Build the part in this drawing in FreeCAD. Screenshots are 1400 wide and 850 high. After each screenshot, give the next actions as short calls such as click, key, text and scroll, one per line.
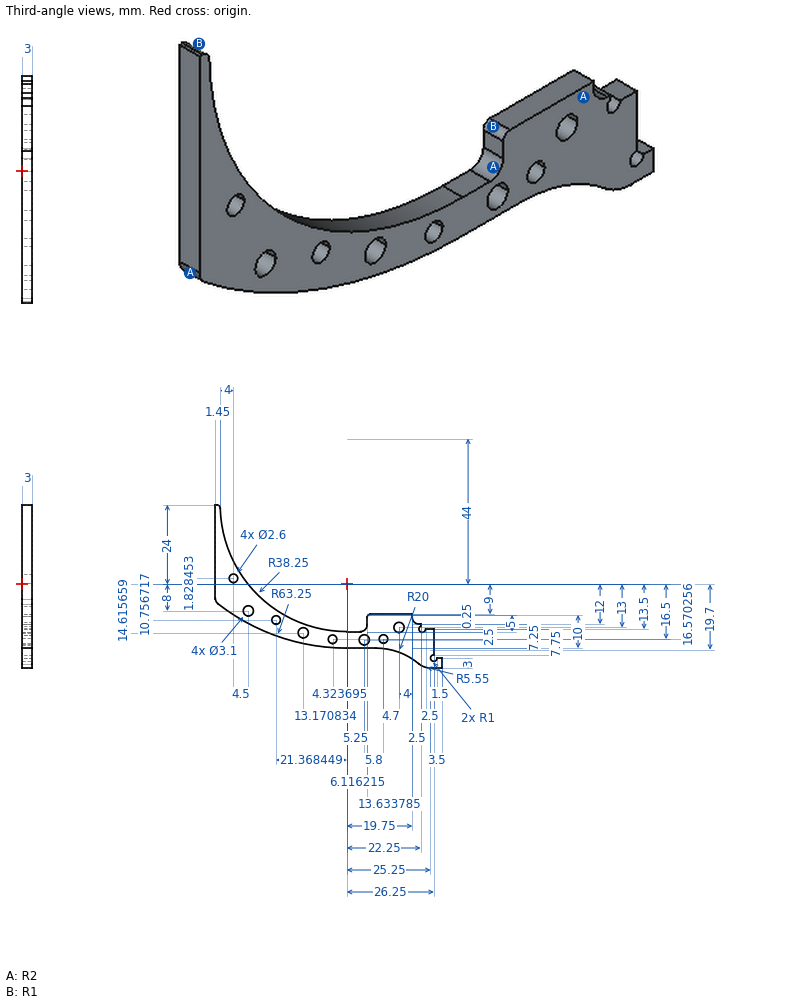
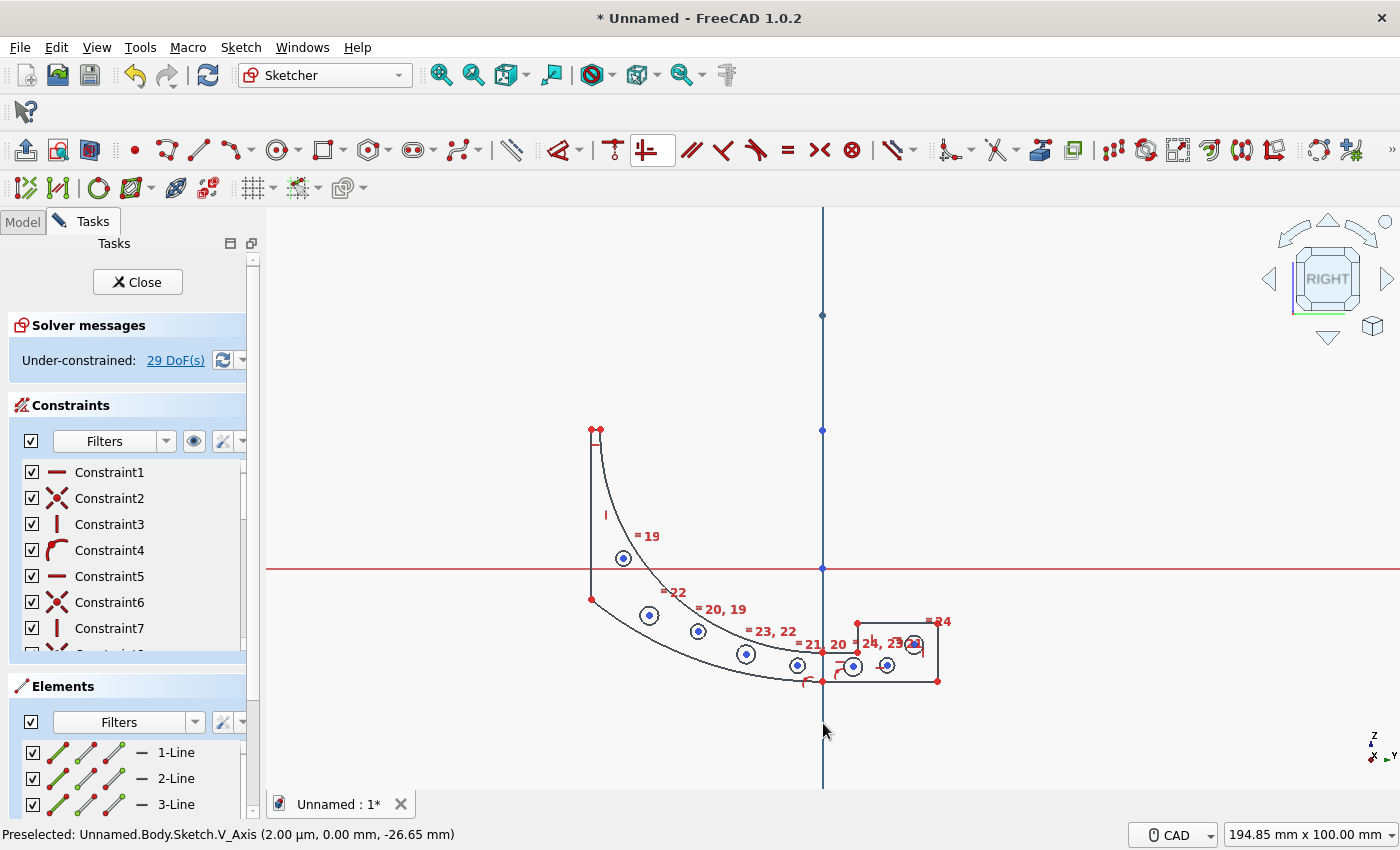
key(c)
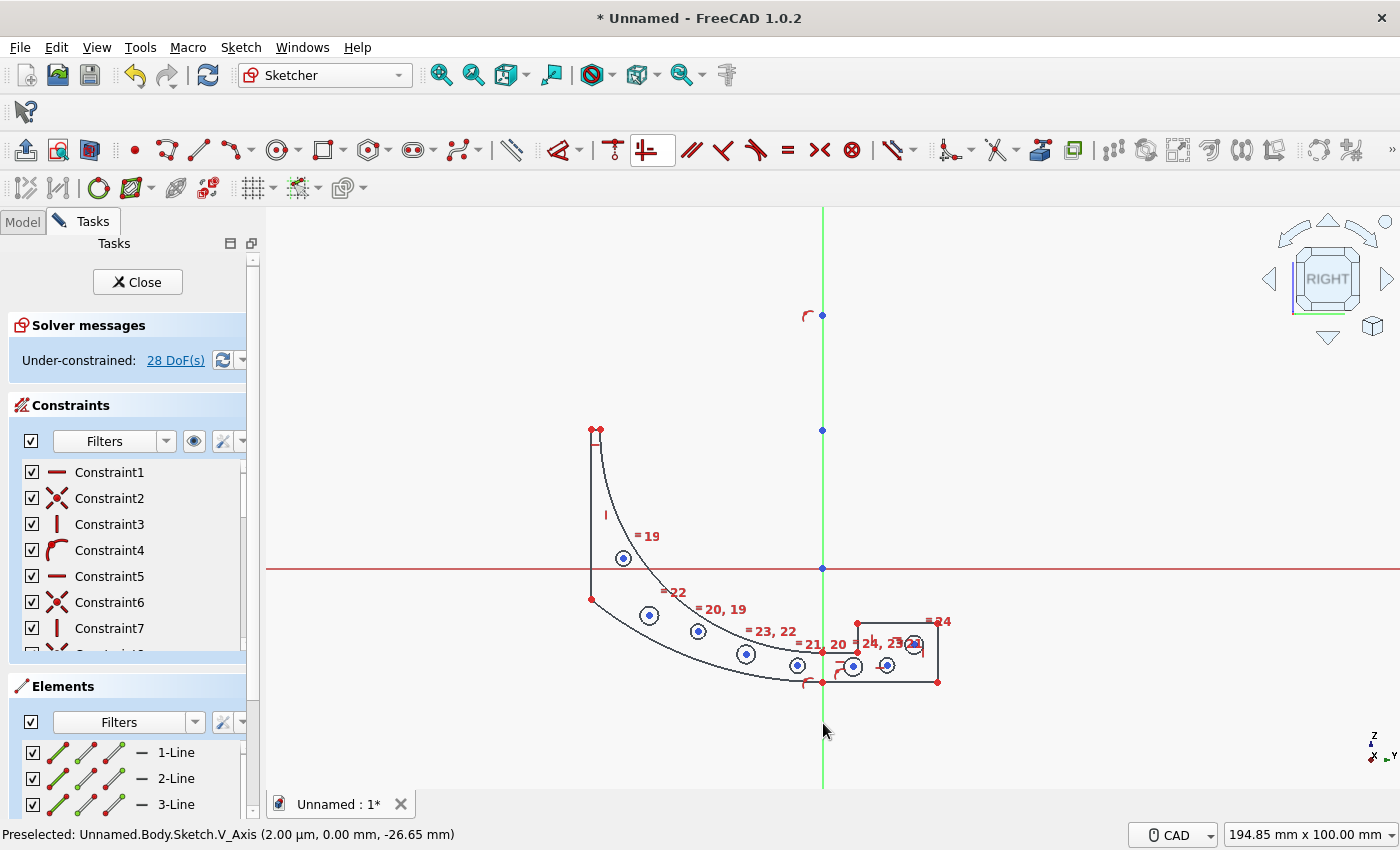
click(823, 430)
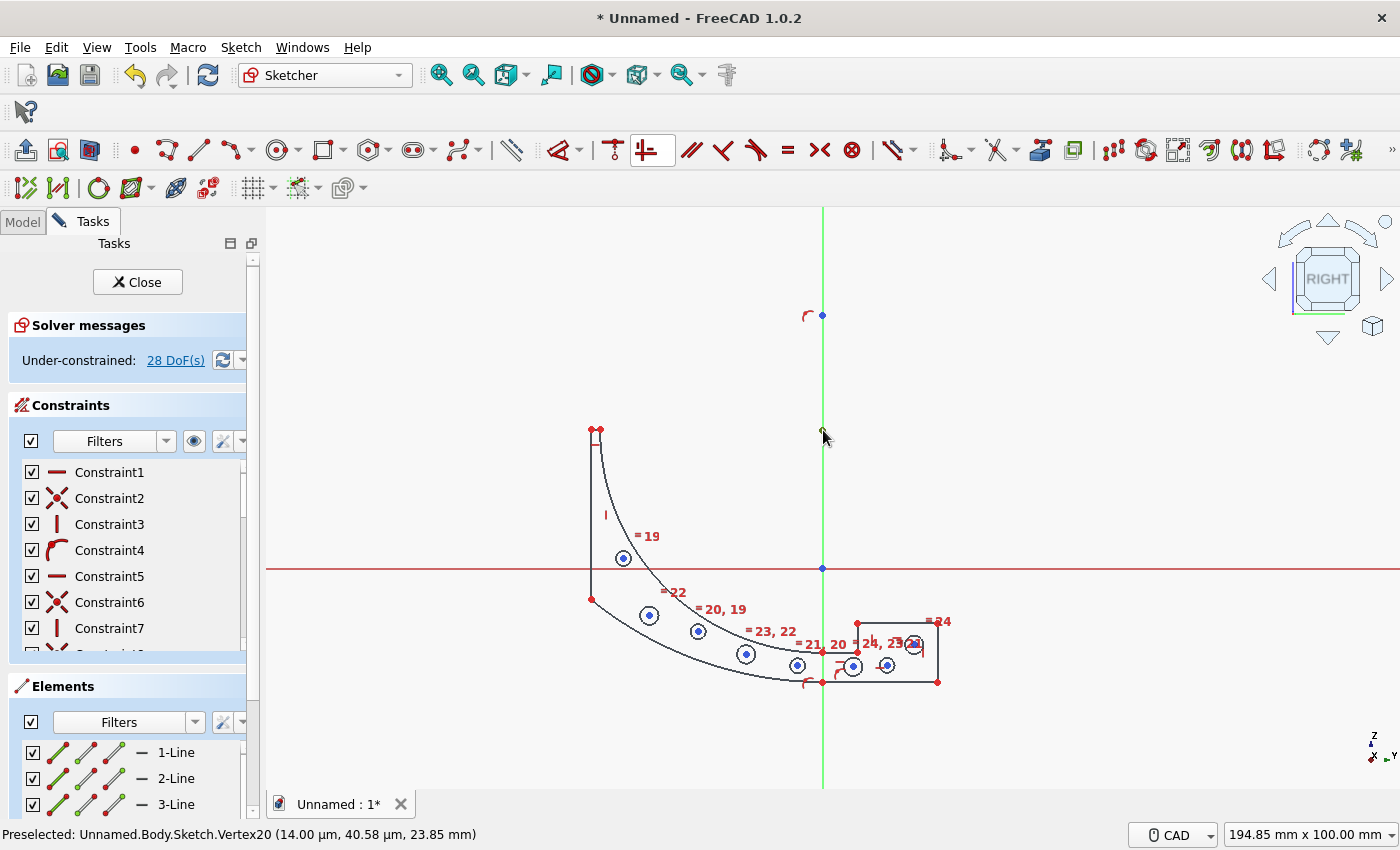
click(823, 723)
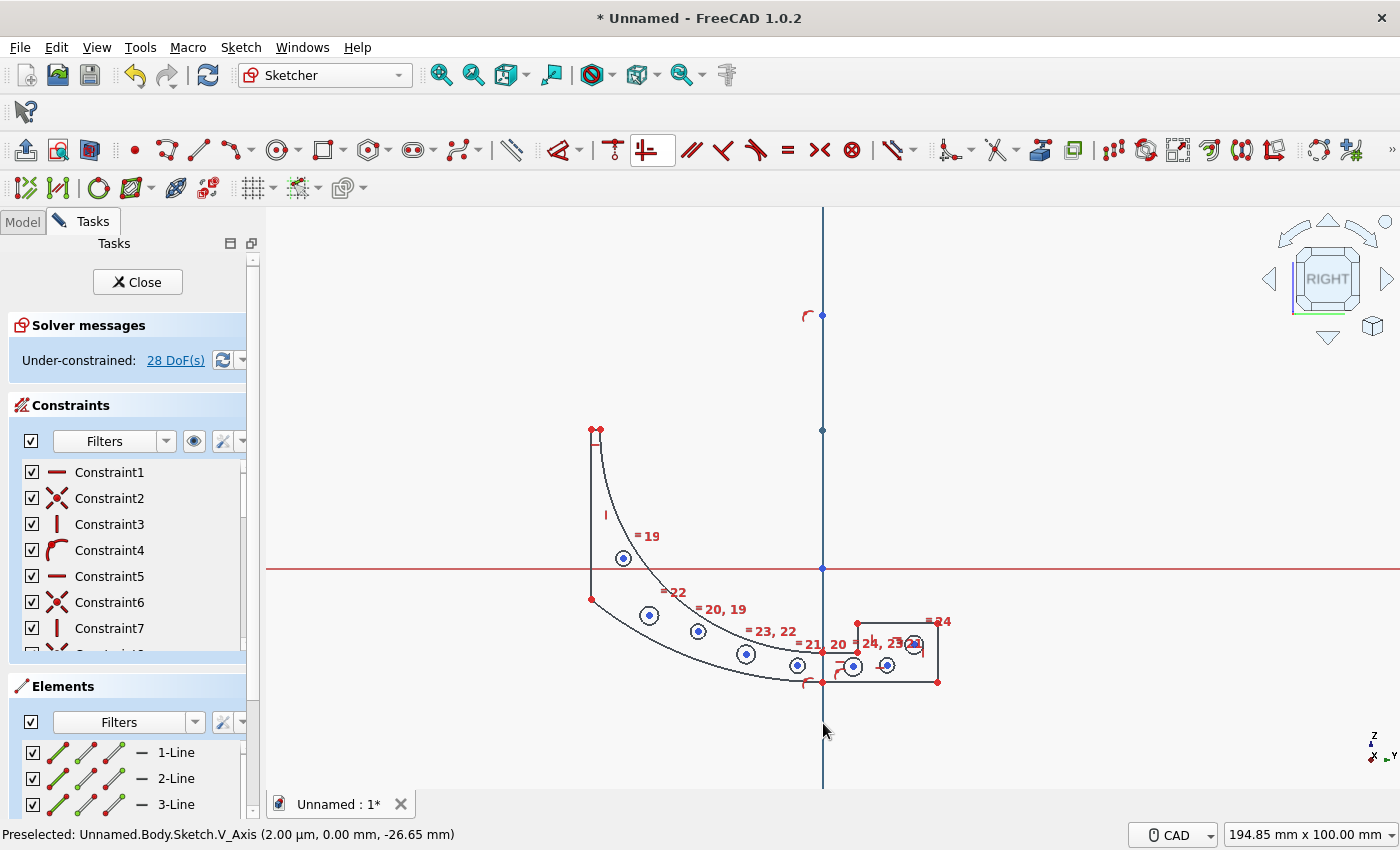
key(c)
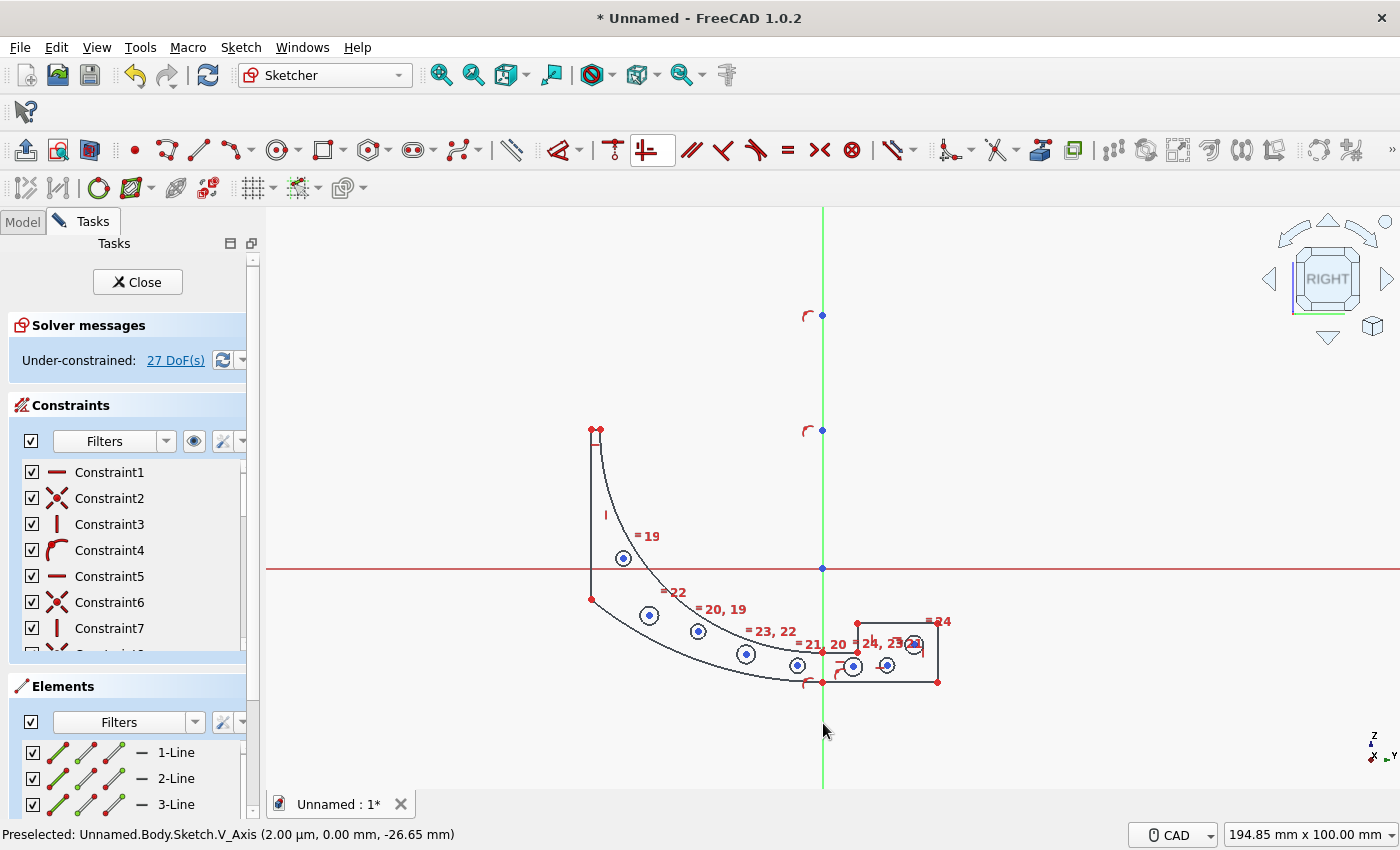
click(558, 150)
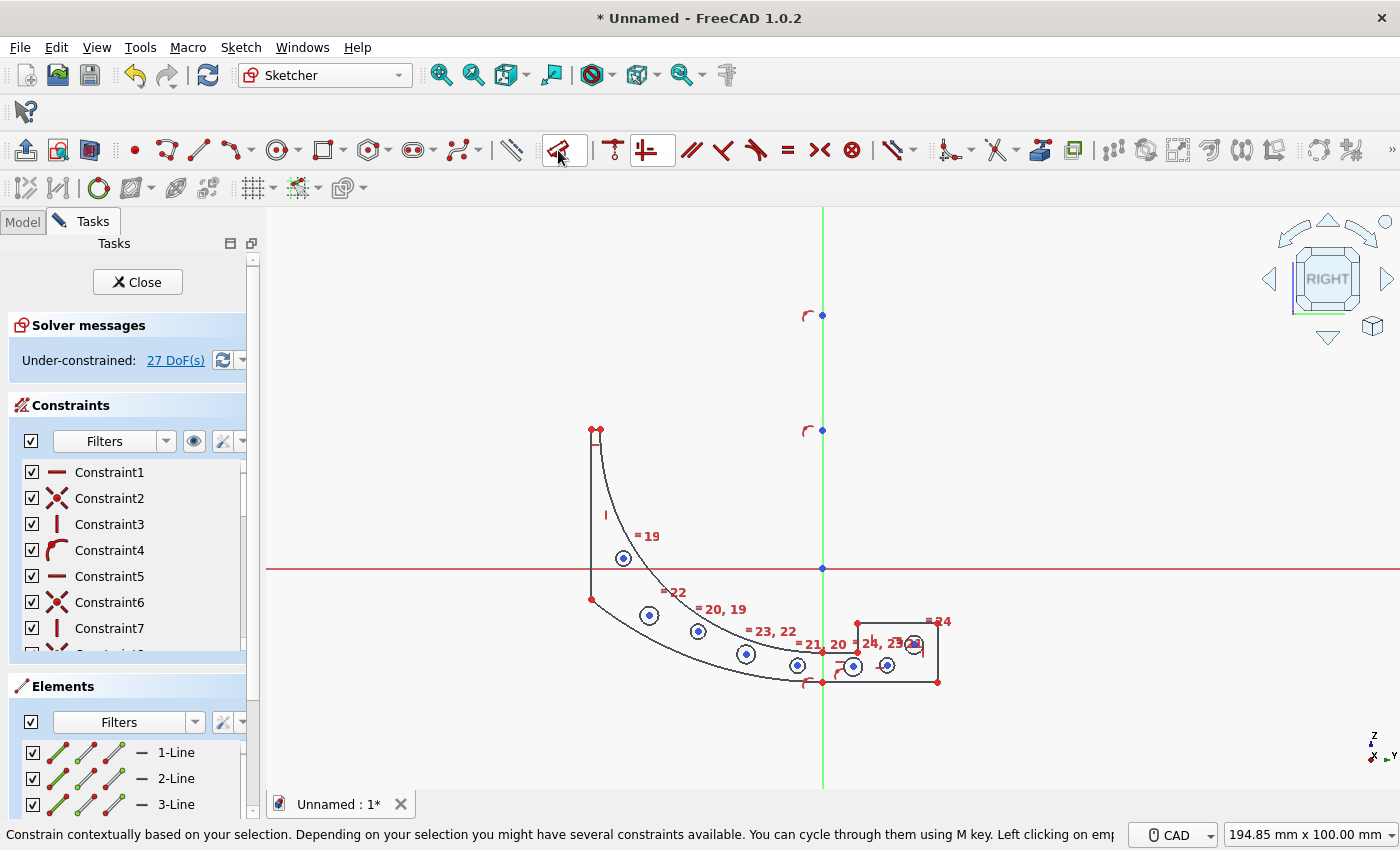
click(654, 641)
click(639, 669)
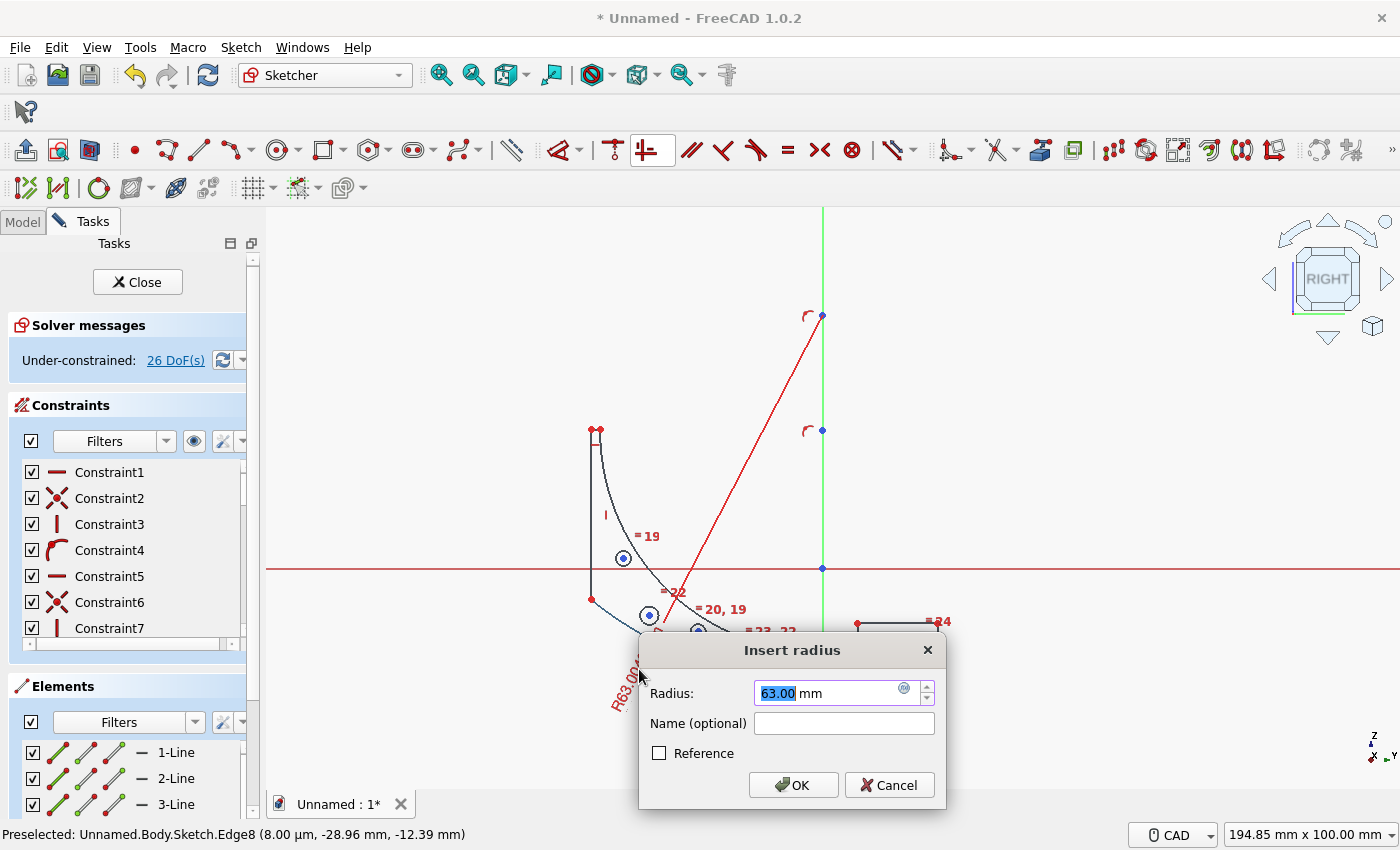
text(63.25)
key(Return)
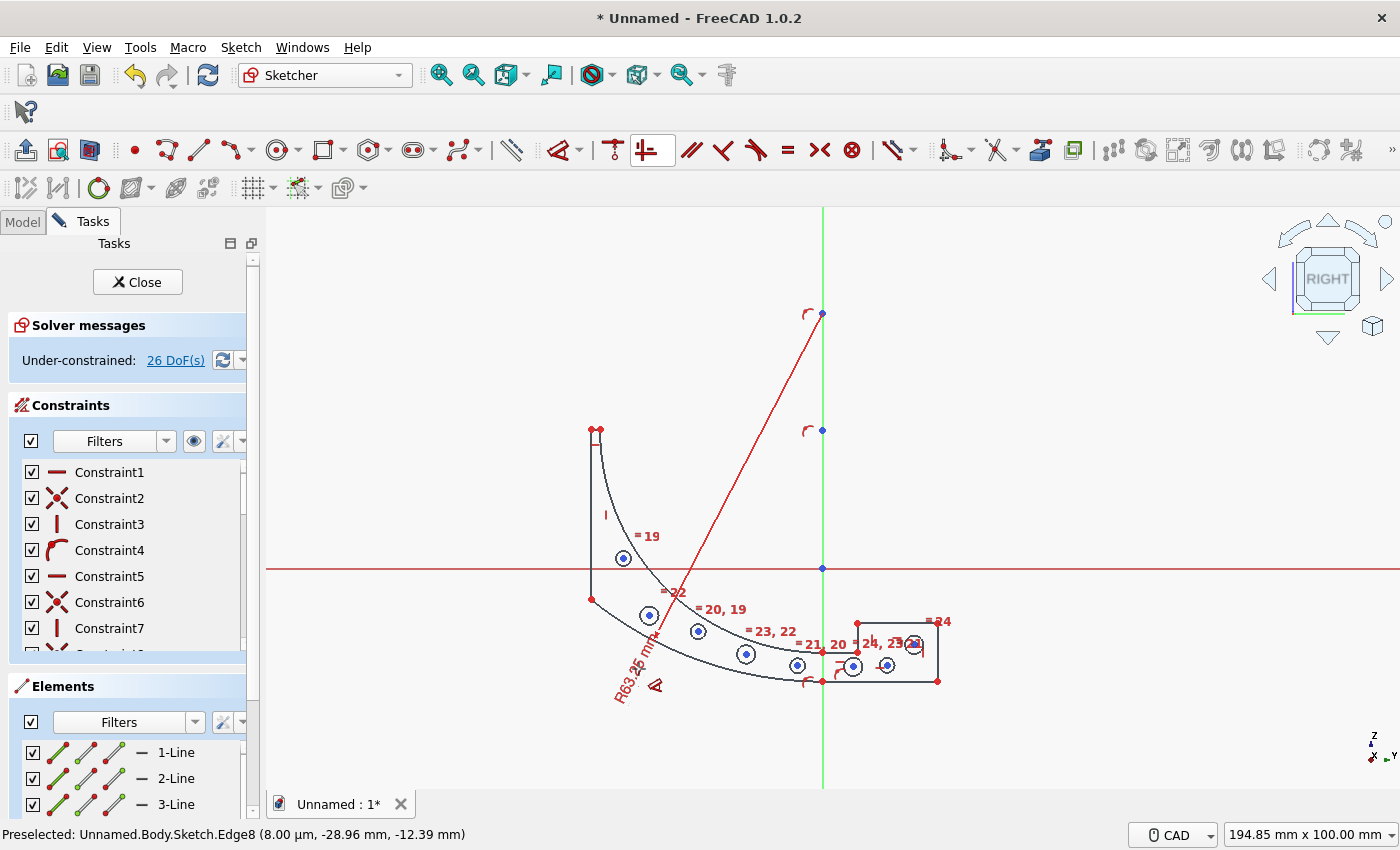
click(624, 531)
click(568, 422)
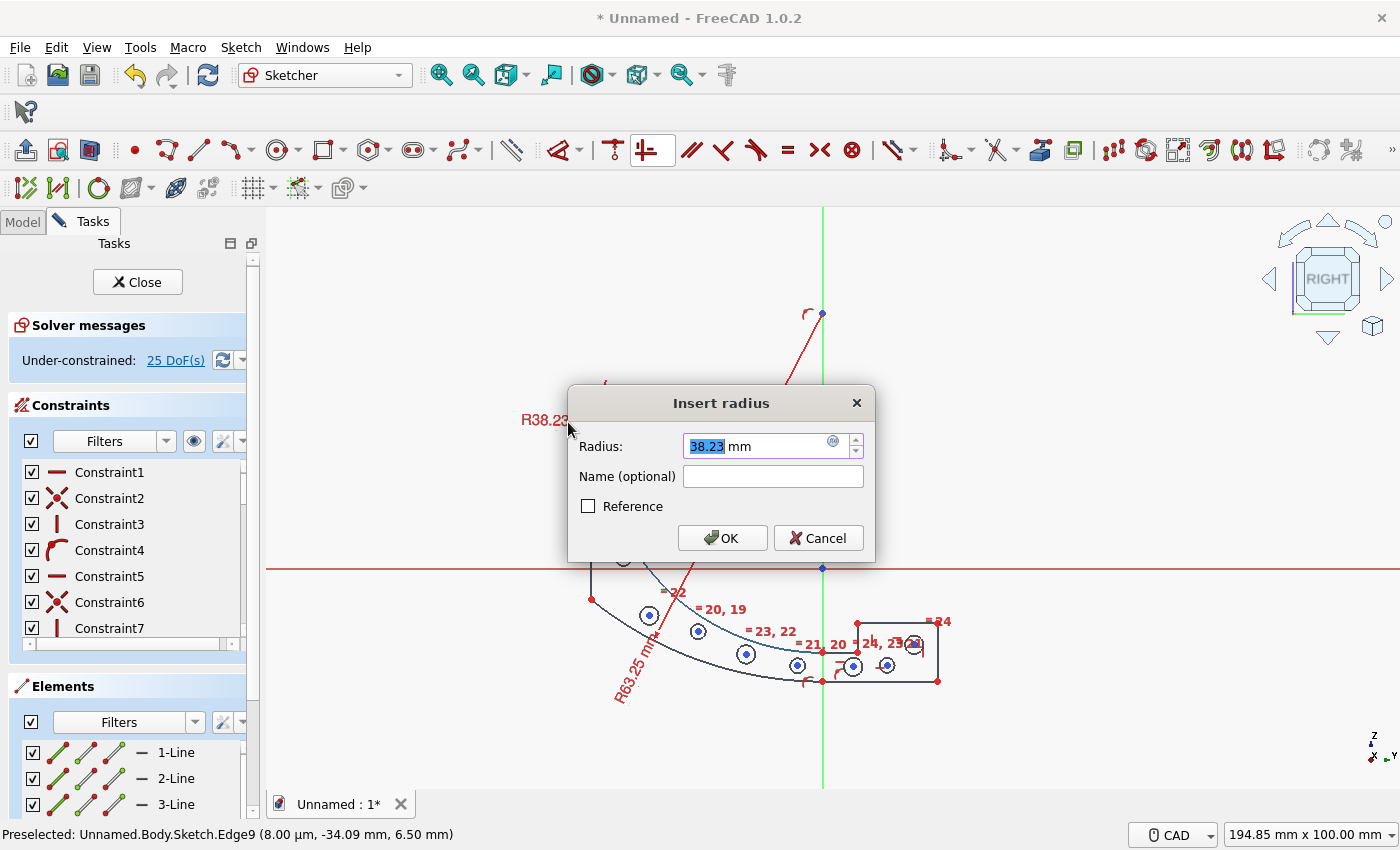
text(38.25)
key(Return)